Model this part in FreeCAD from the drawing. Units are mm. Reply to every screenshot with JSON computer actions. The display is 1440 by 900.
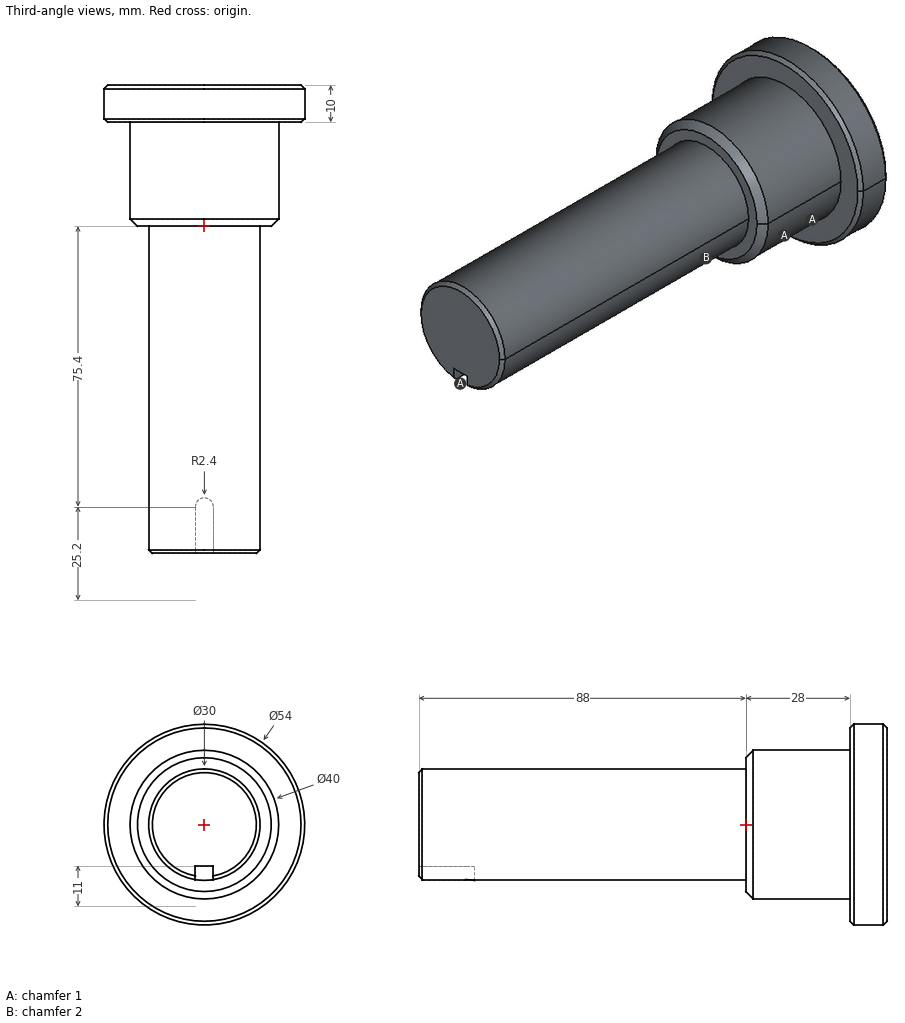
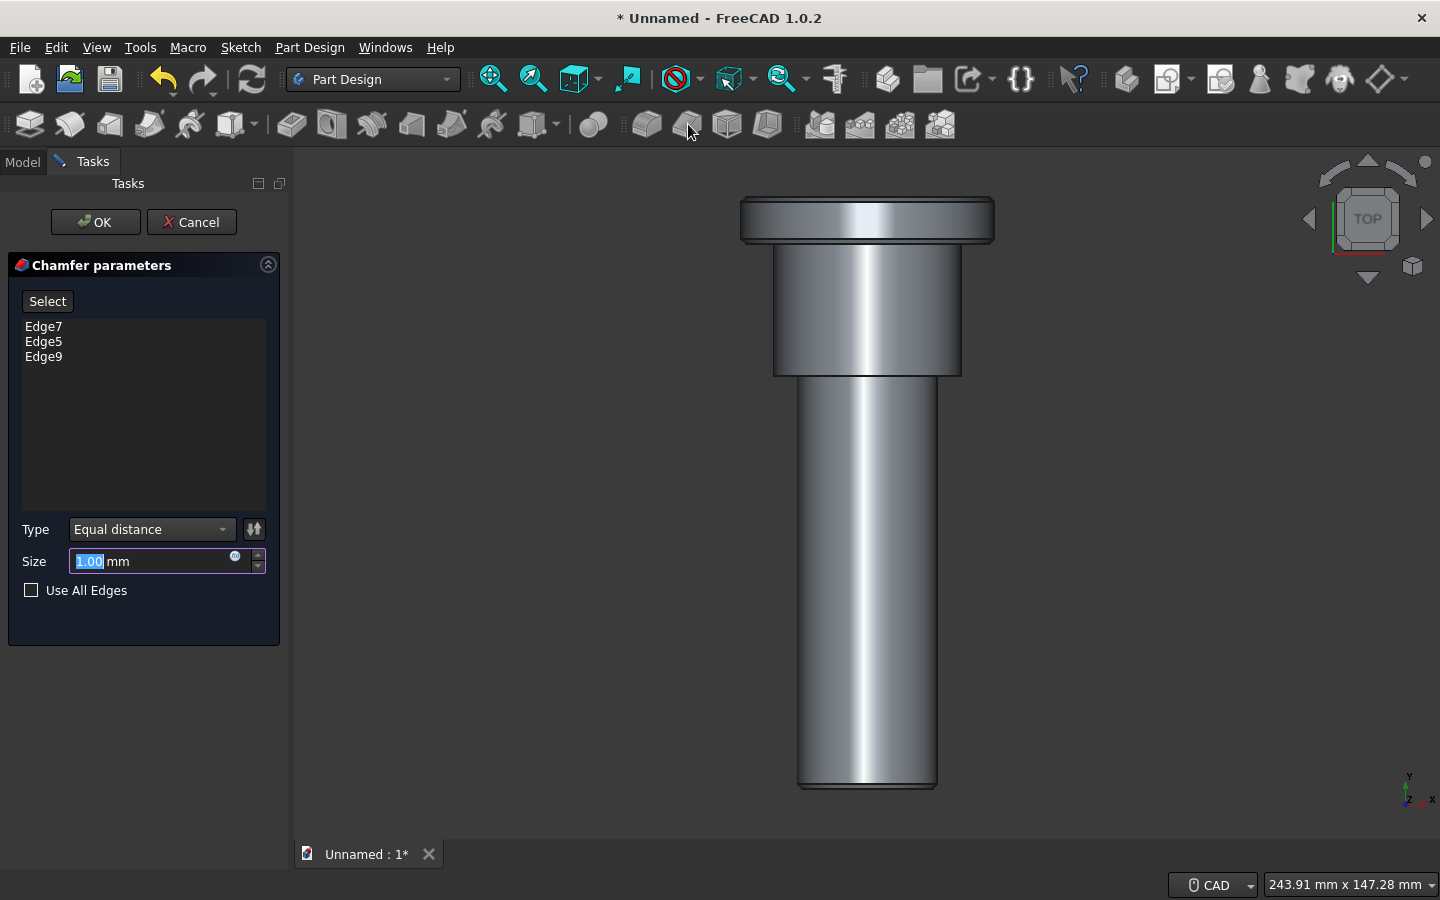
{"action": "type", "text": "1"}
{"action": "key", "text": "Tab"}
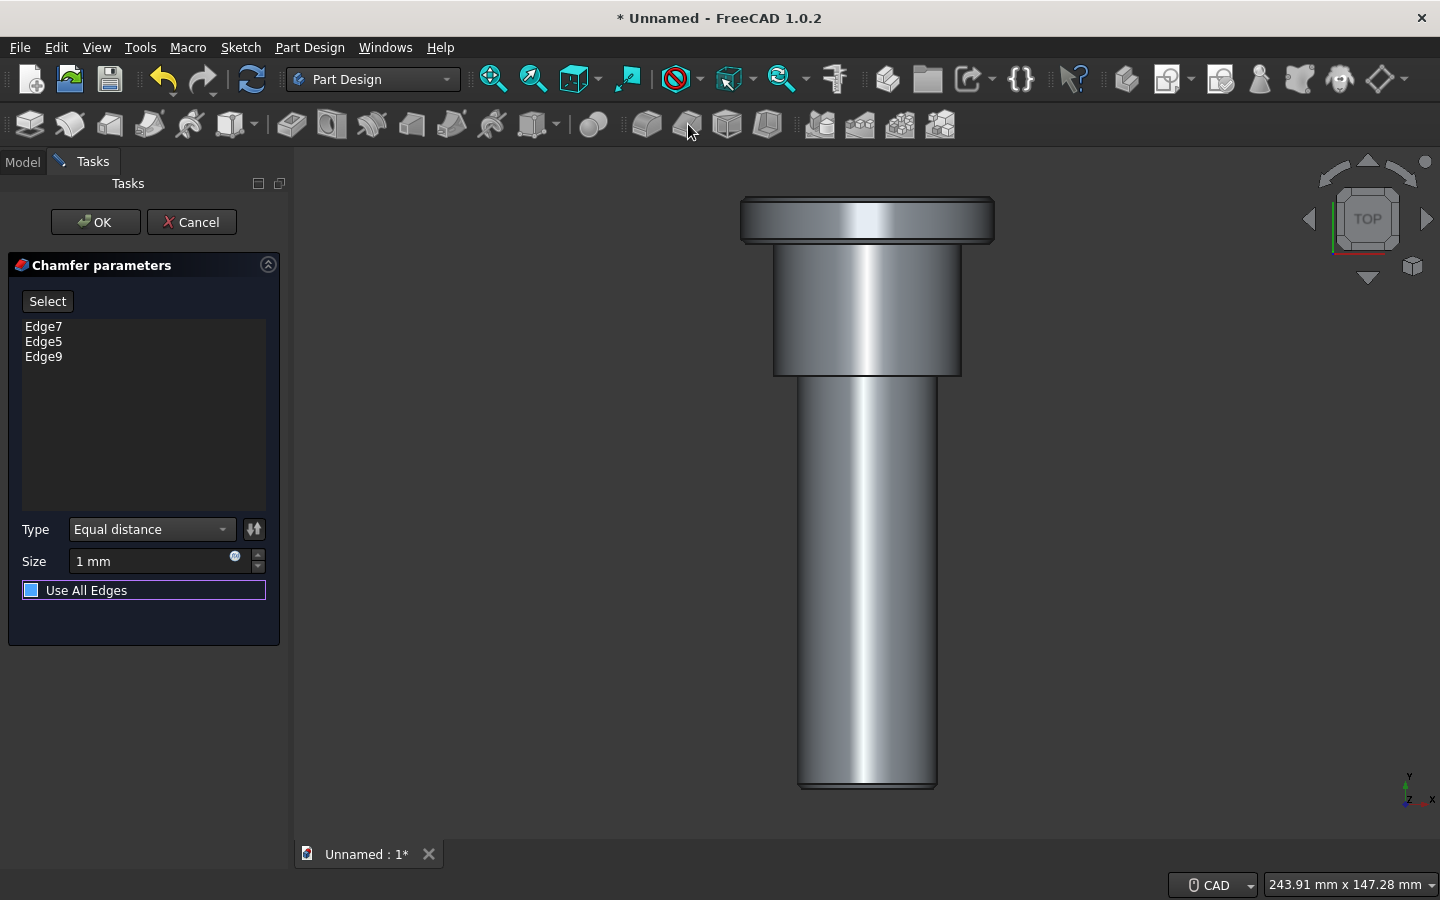
{"action": "left_click", "coordinate": [96, 222]}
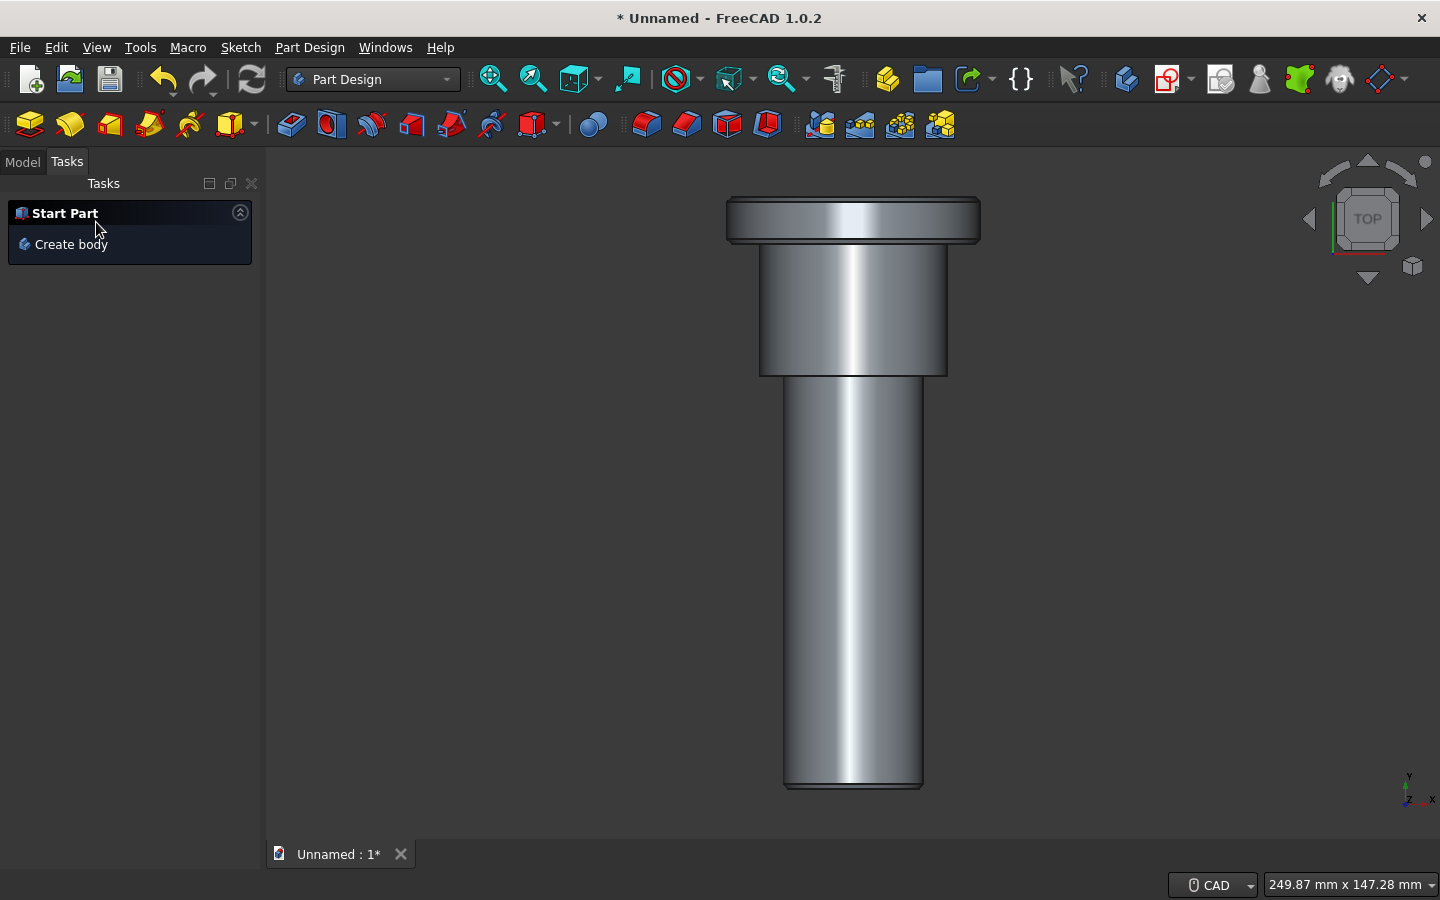
{"action": "key", "text": "0"}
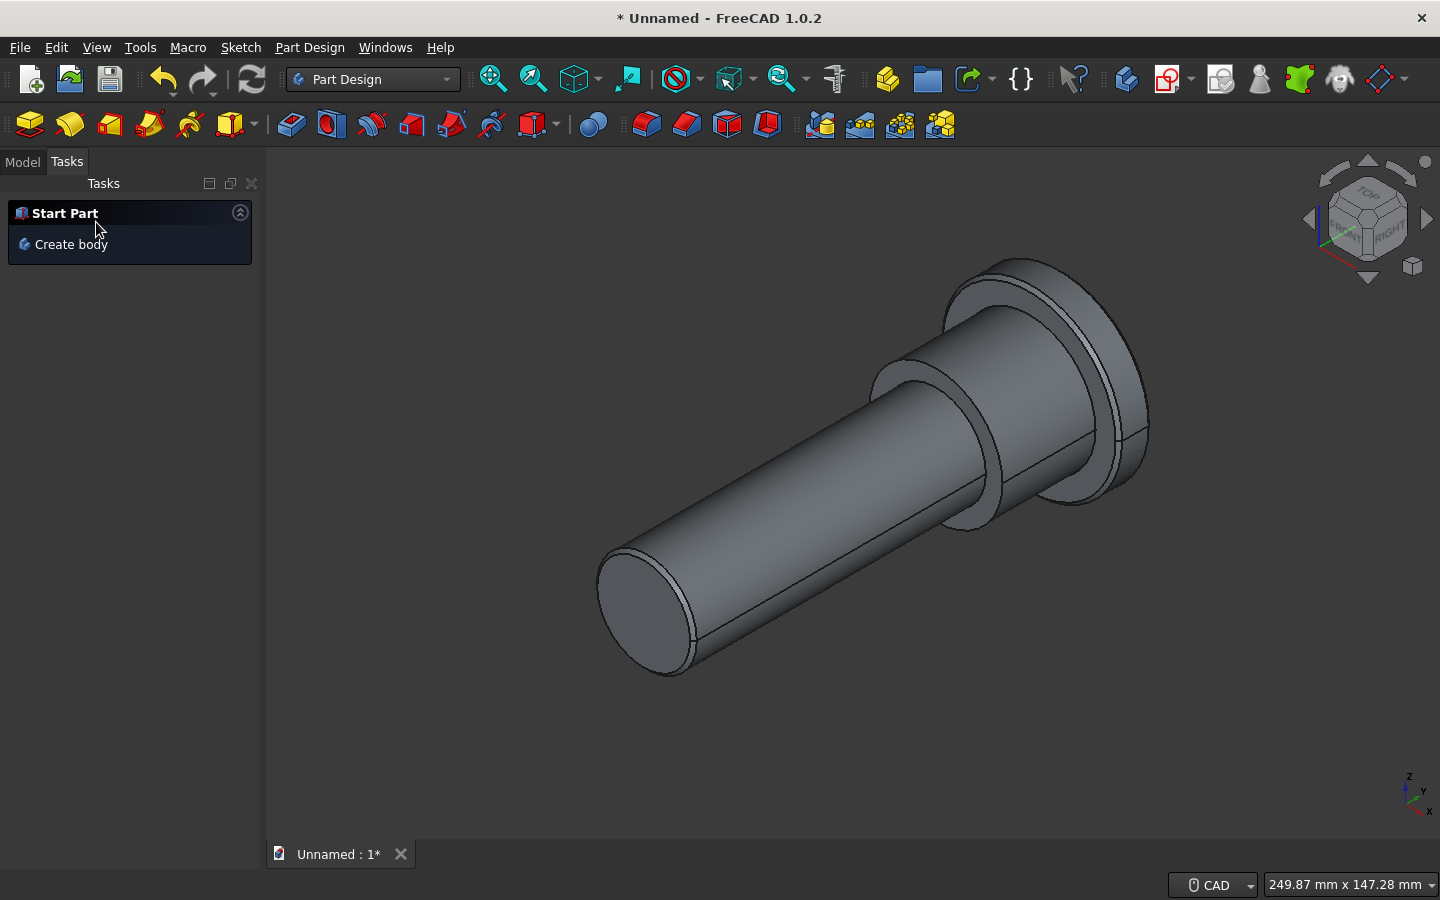
{"action": "left_click", "coordinate": [916, 359]}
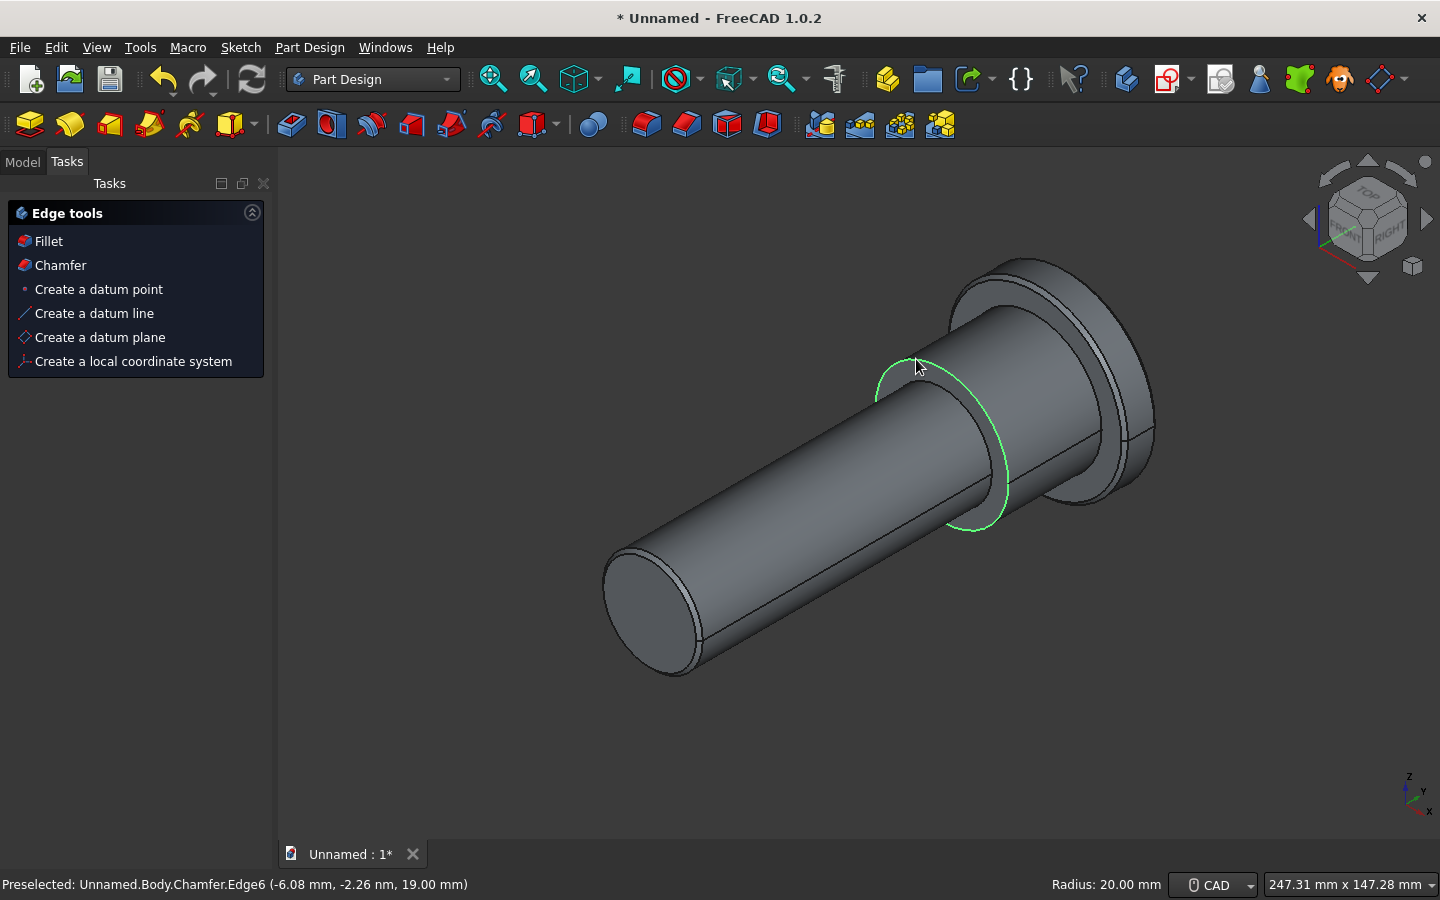
{"action": "left_click", "coordinate": [688, 124]}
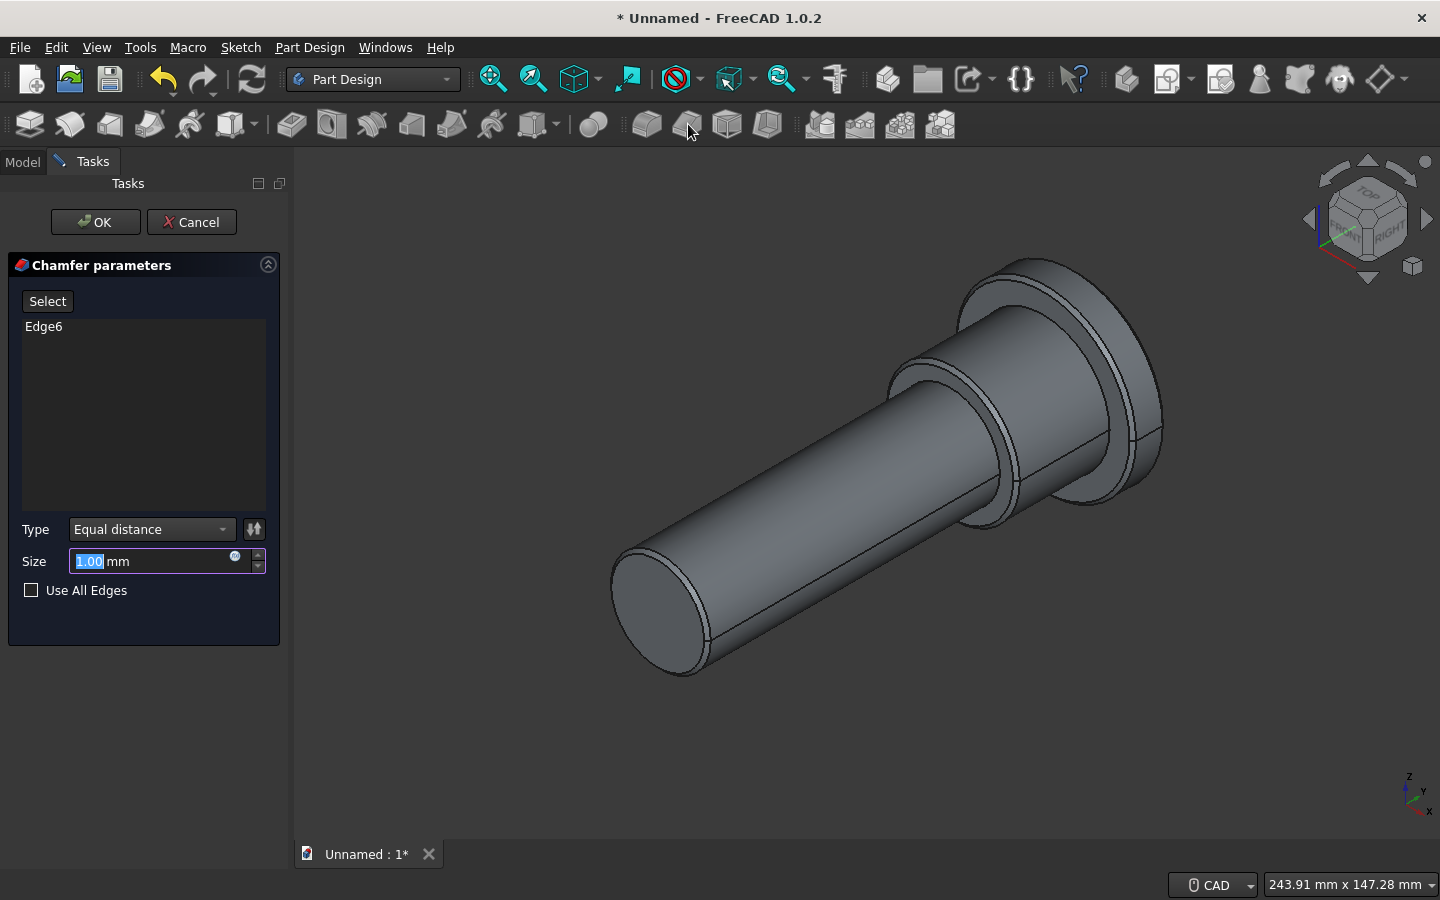
{"action": "type", "text": "2"}
{"action": "key", "text": "Tab"}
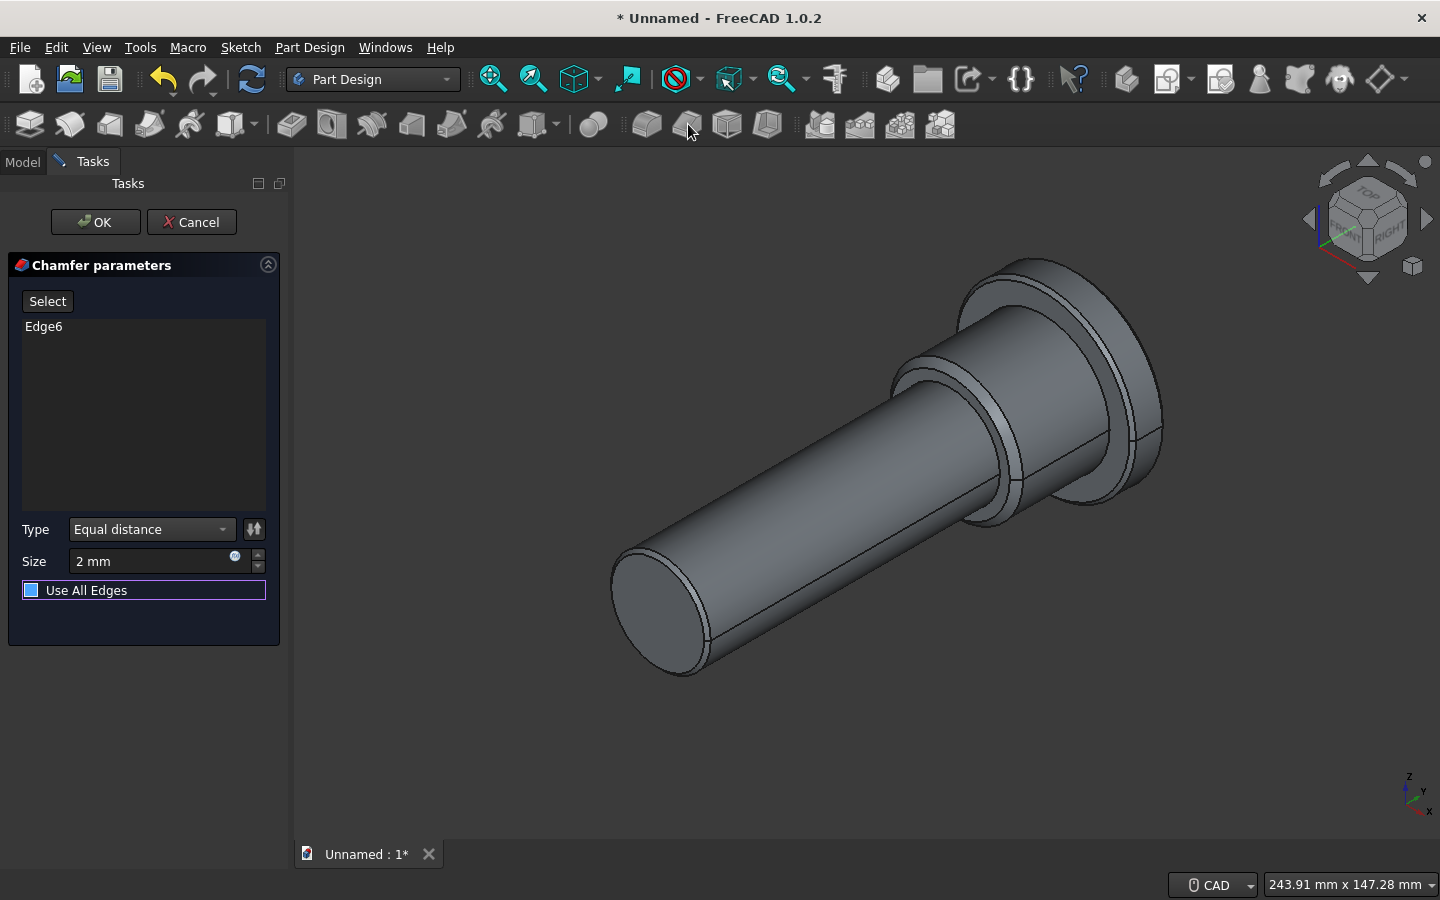
{"action": "left_click", "coordinate": [96, 222]}